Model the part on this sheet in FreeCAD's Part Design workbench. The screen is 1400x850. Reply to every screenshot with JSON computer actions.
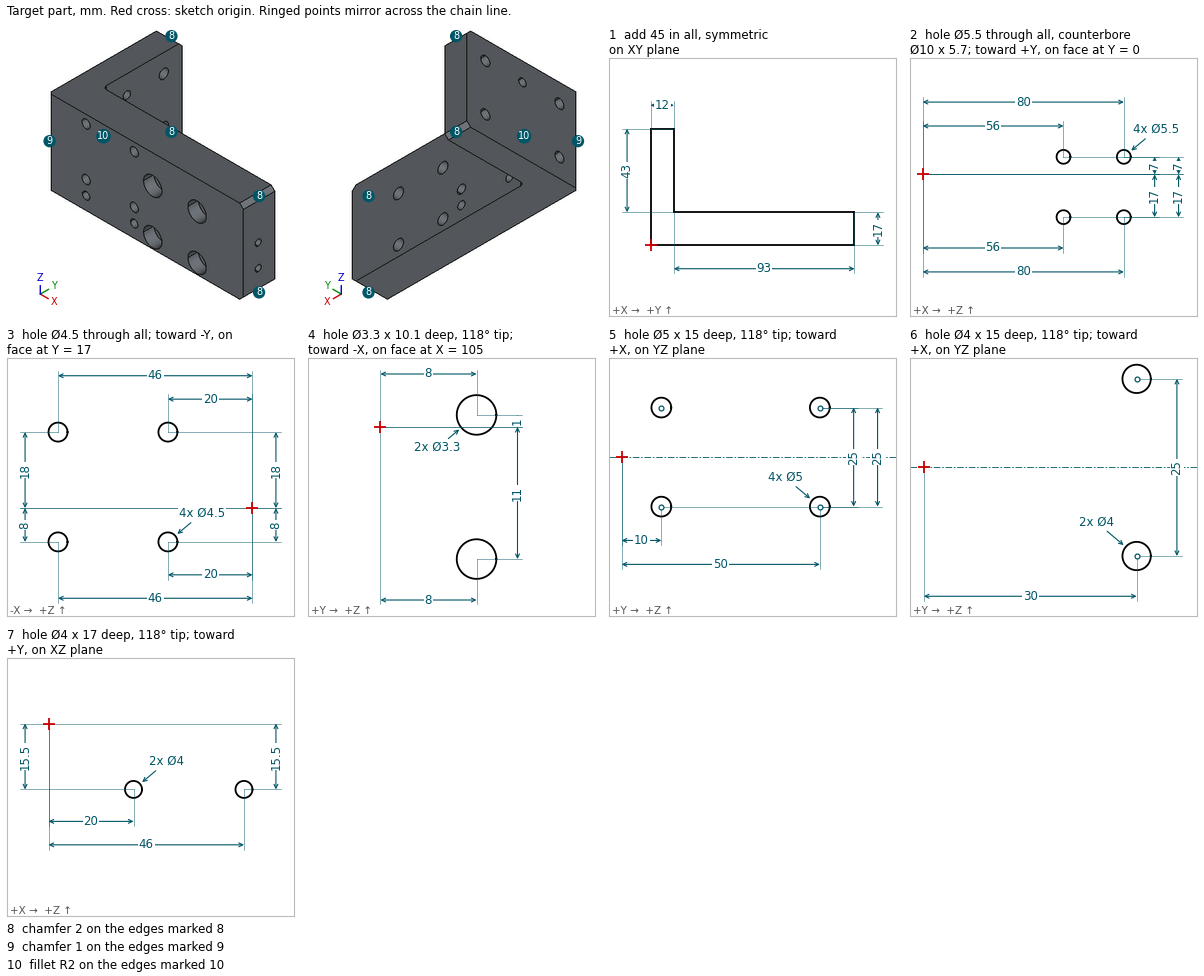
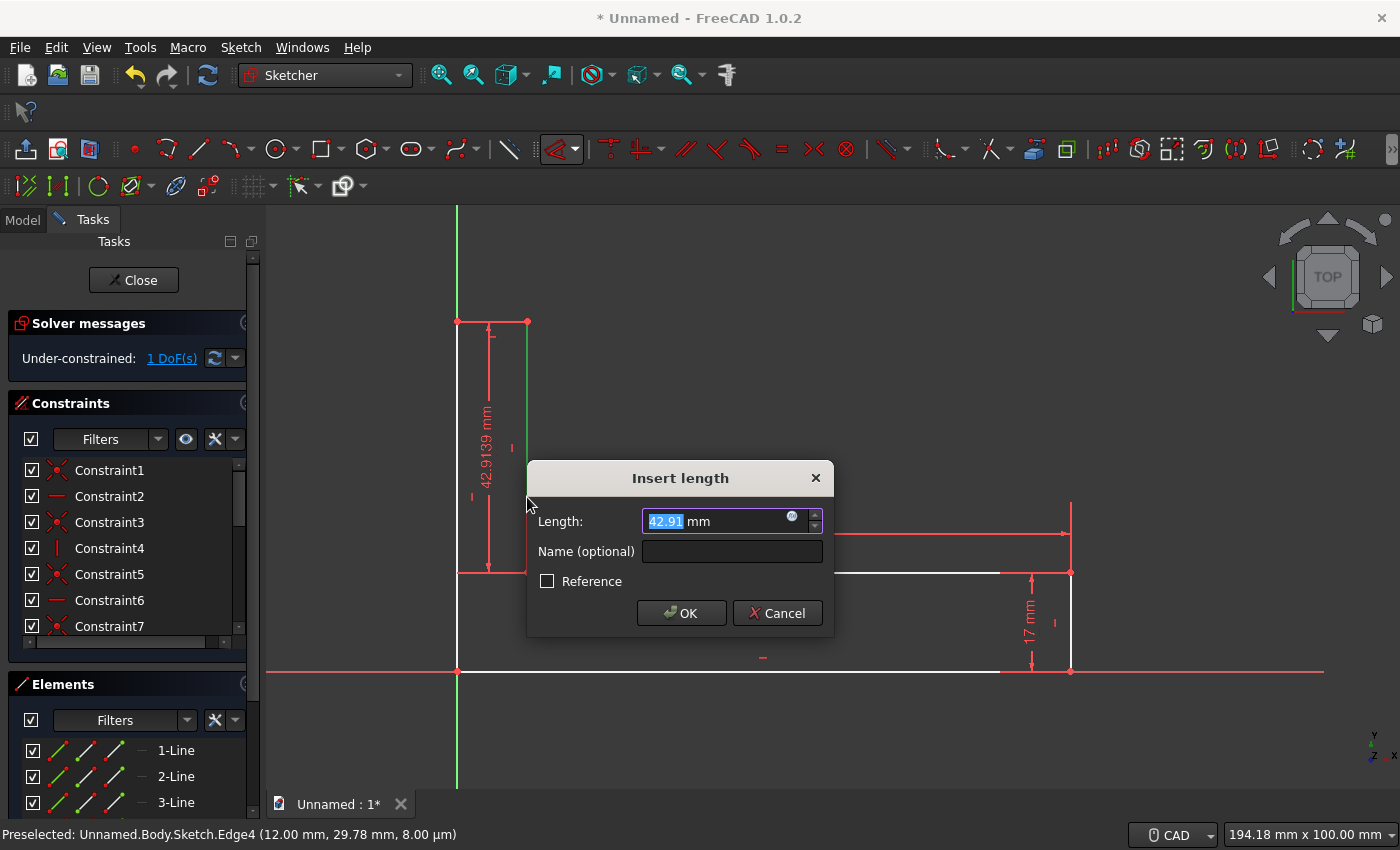
{"action": "type", "text": "43"}
{"action": "key", "text": "Return"}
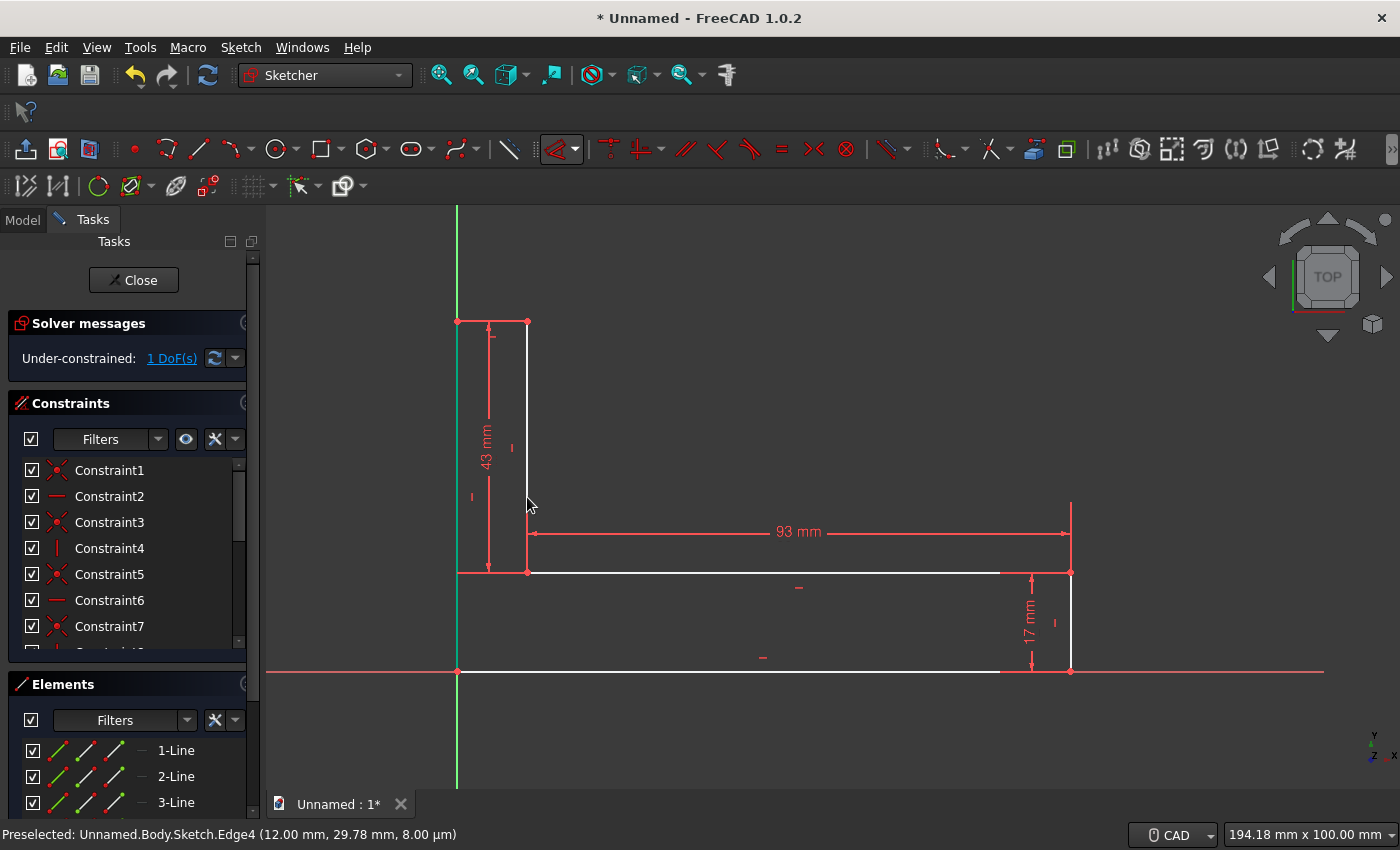
{"action": "left_click", "coordinate": [506, 321]}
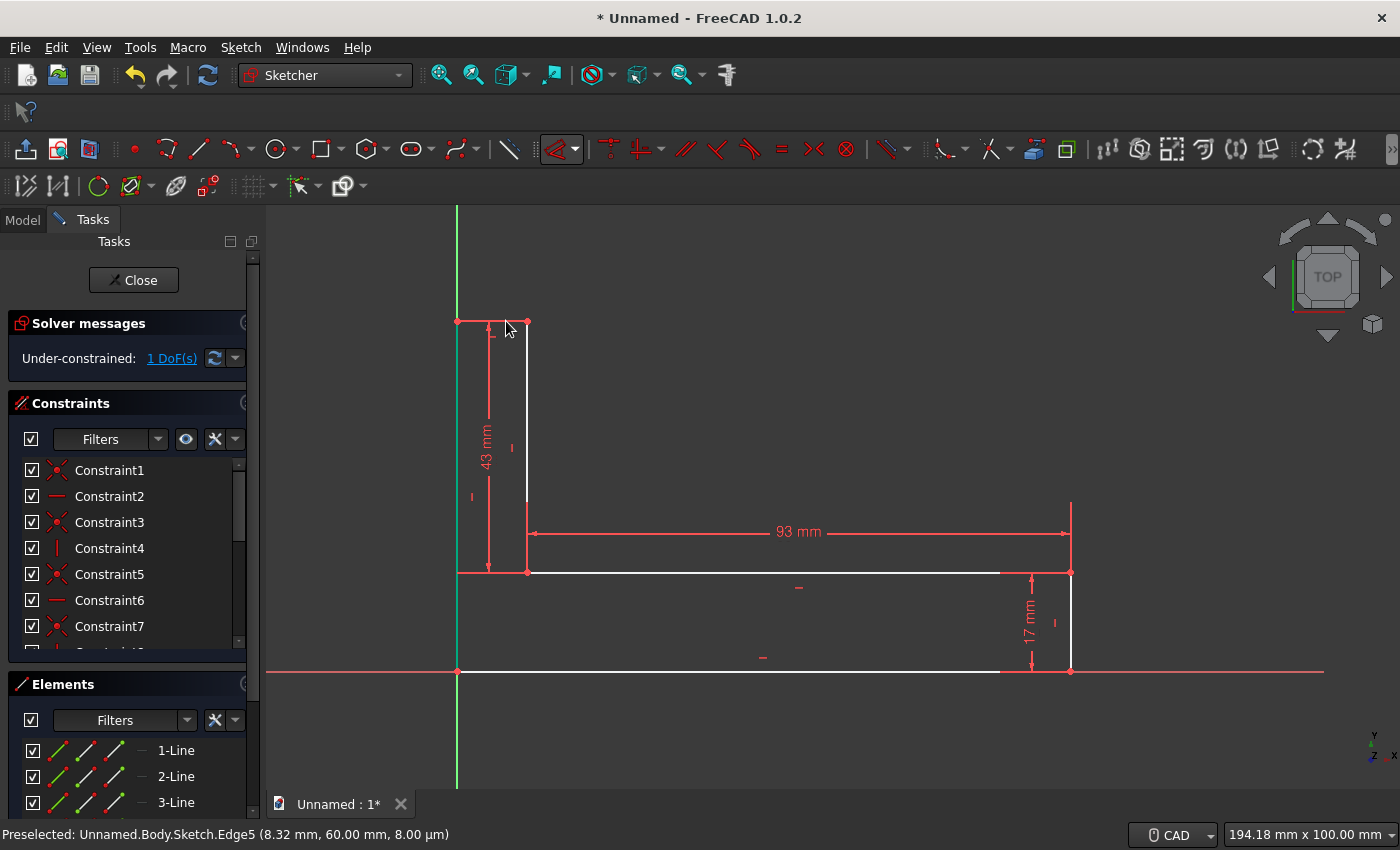
{"action": "key", "text": "l"}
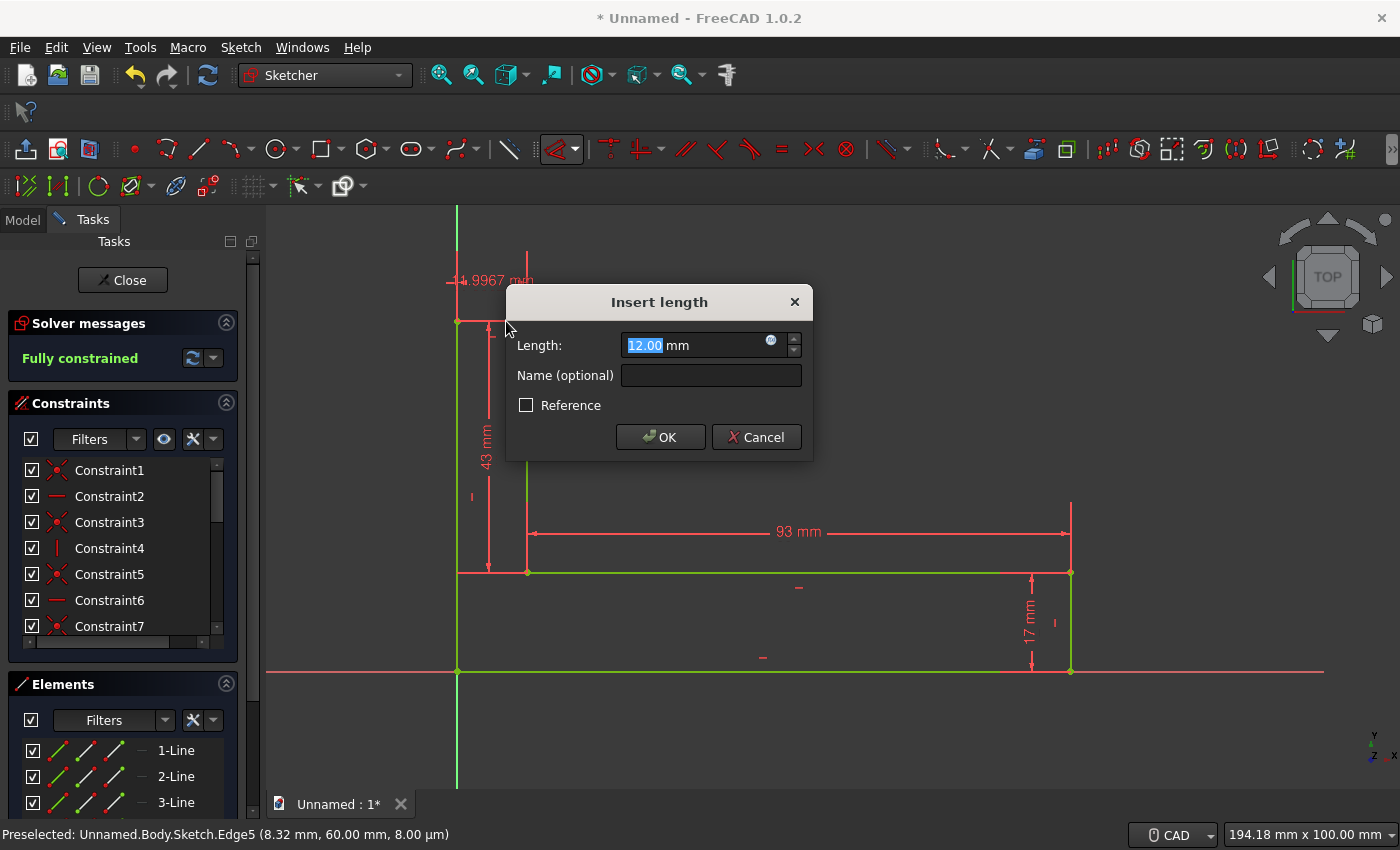
{"action": "type", "text": "12"}
{"action": "key", "text": "Return"}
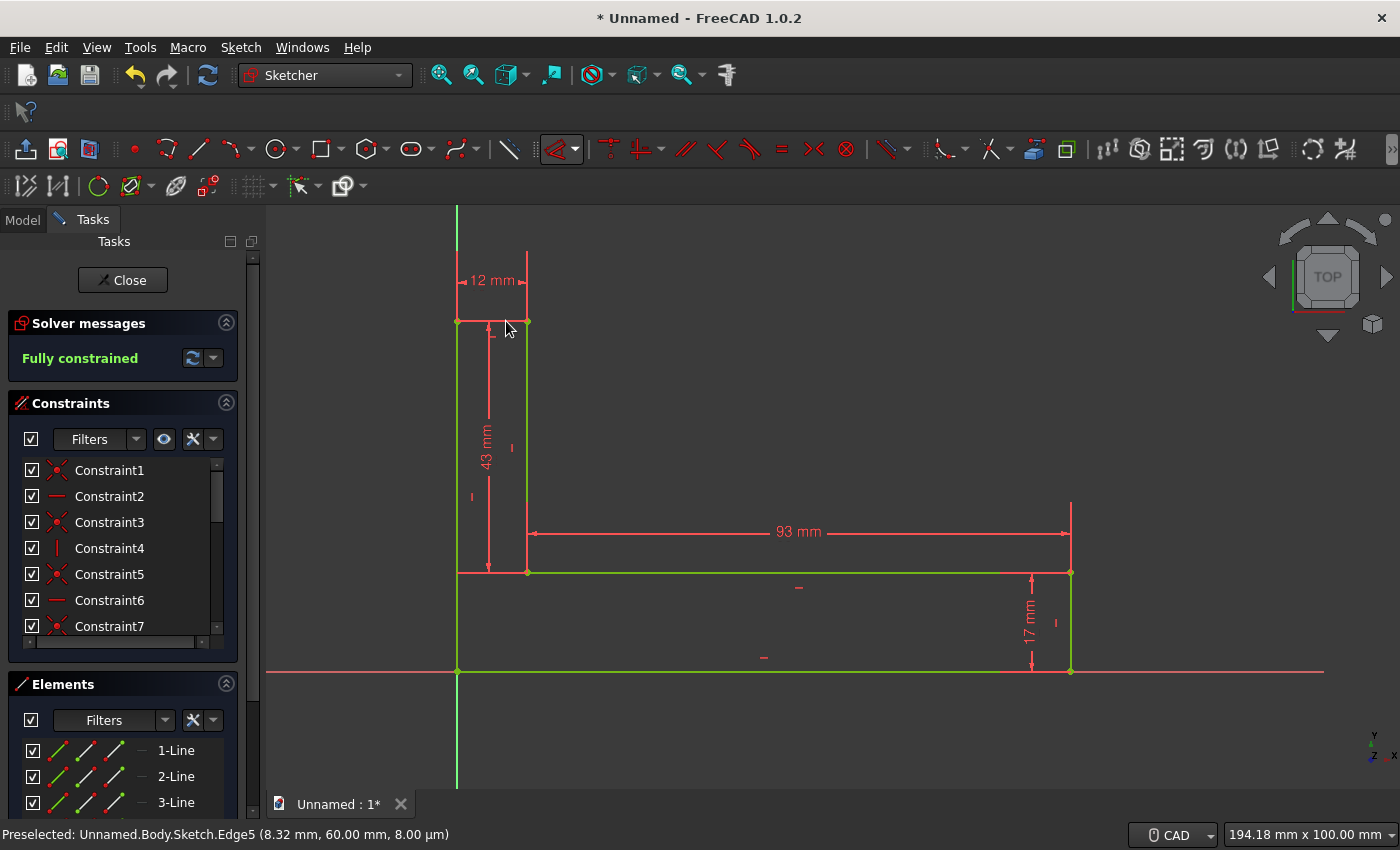
{"action": "left_click", "coordinate": [123, 280]}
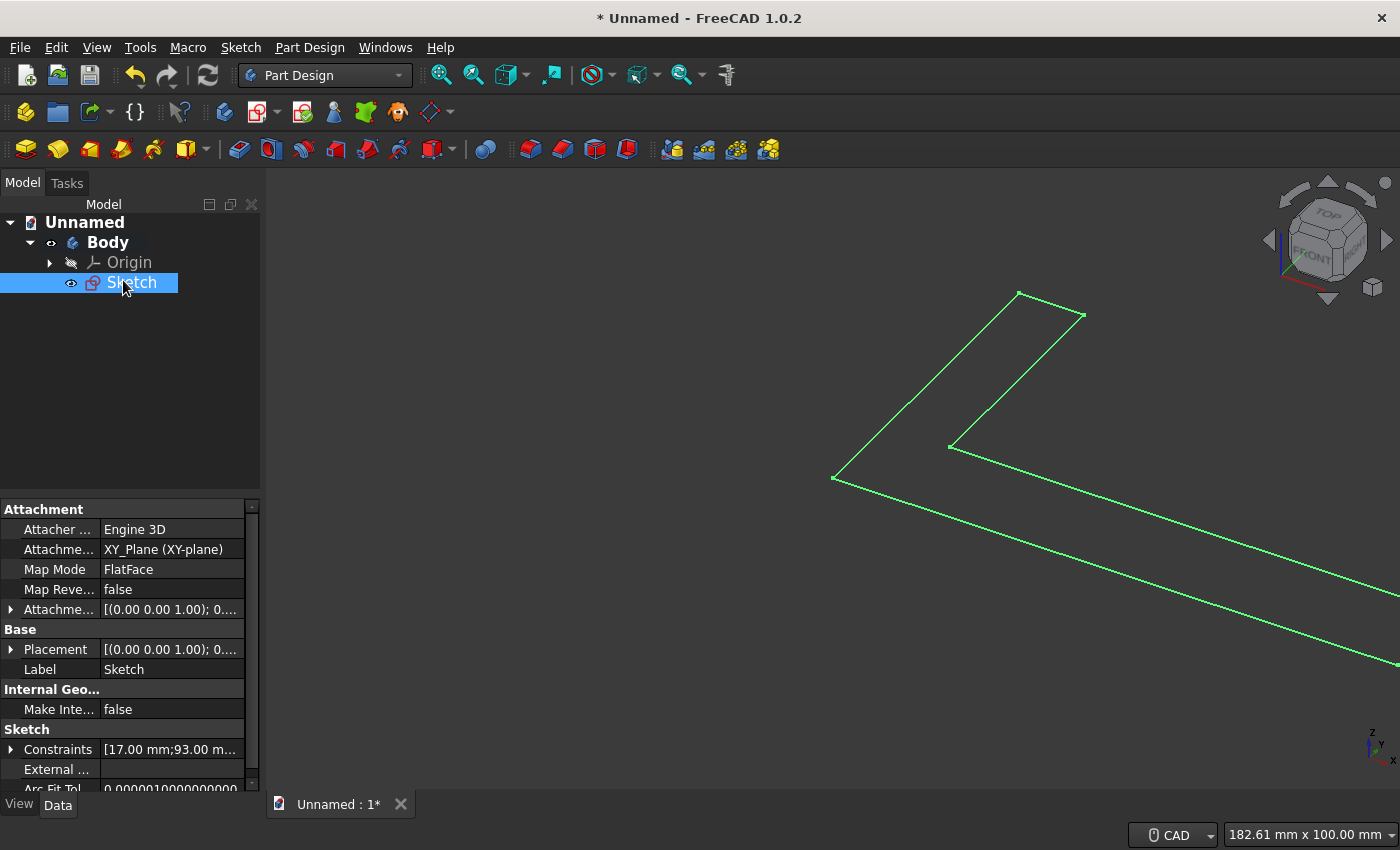
{"action": "left_click", "coordinate": [26, 150]}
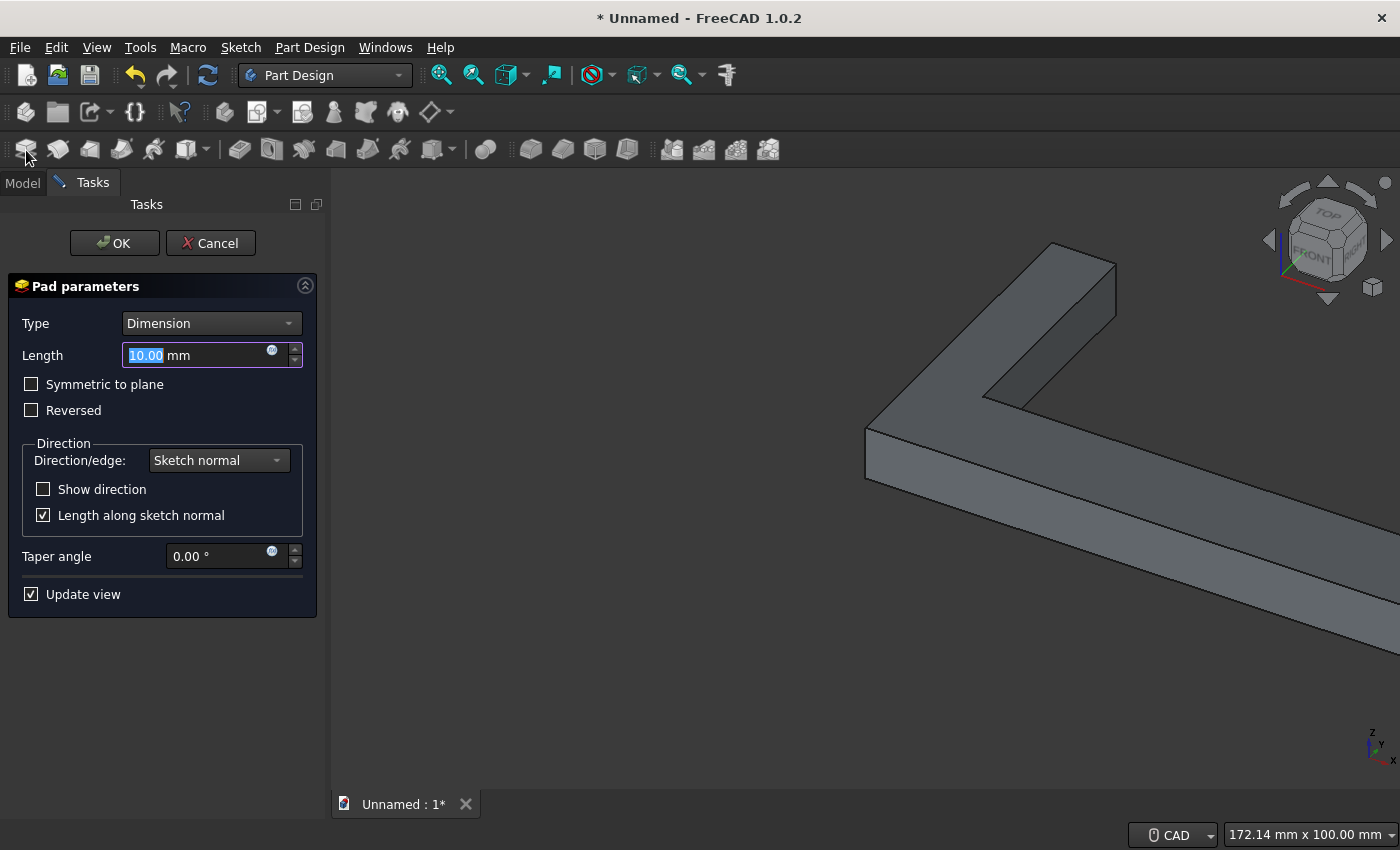
{"action": "type", "text": "45"}
{"action": "key", "text": "Tab"}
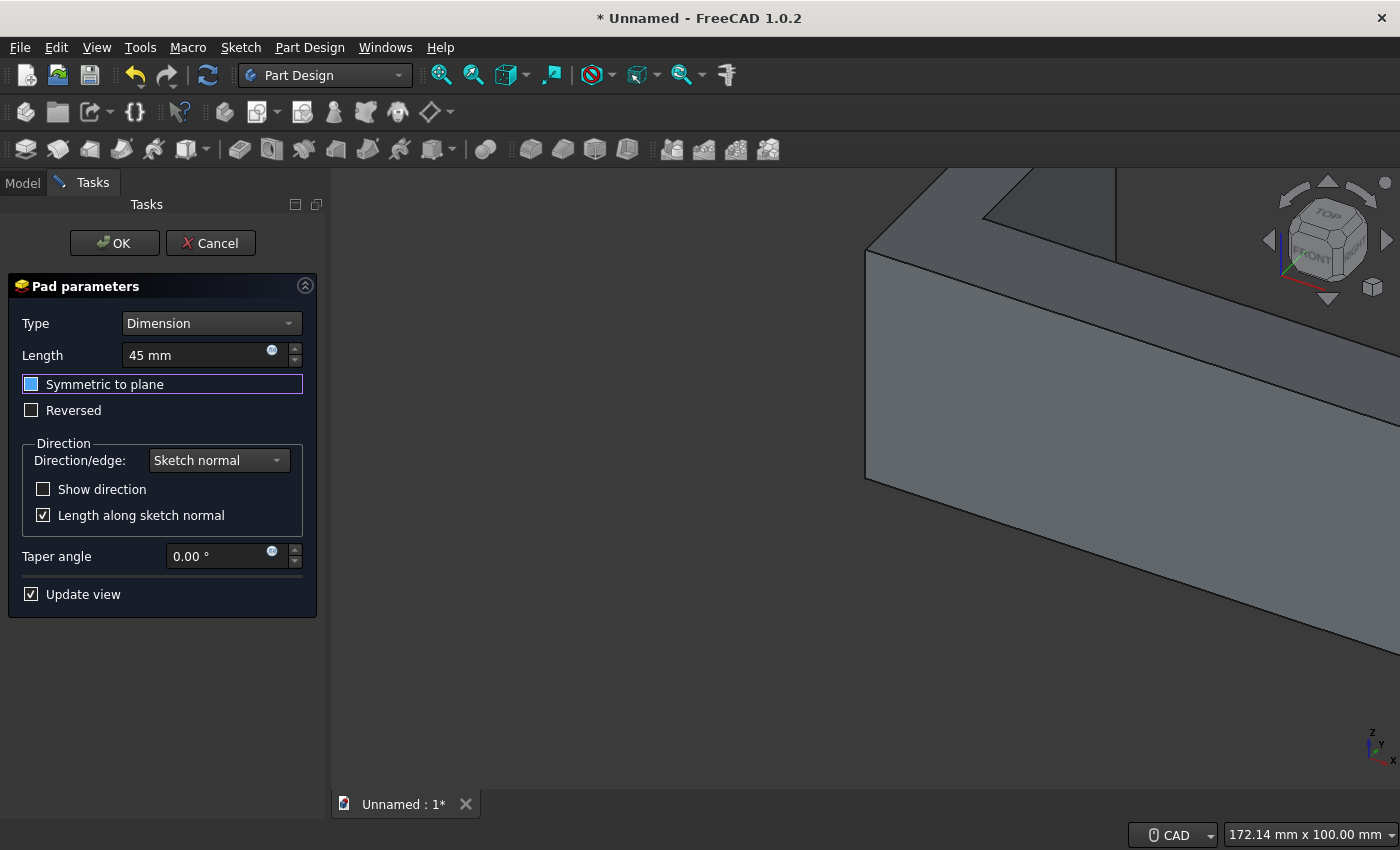
{"action": "left_click", "coordinate": [30, 384]}